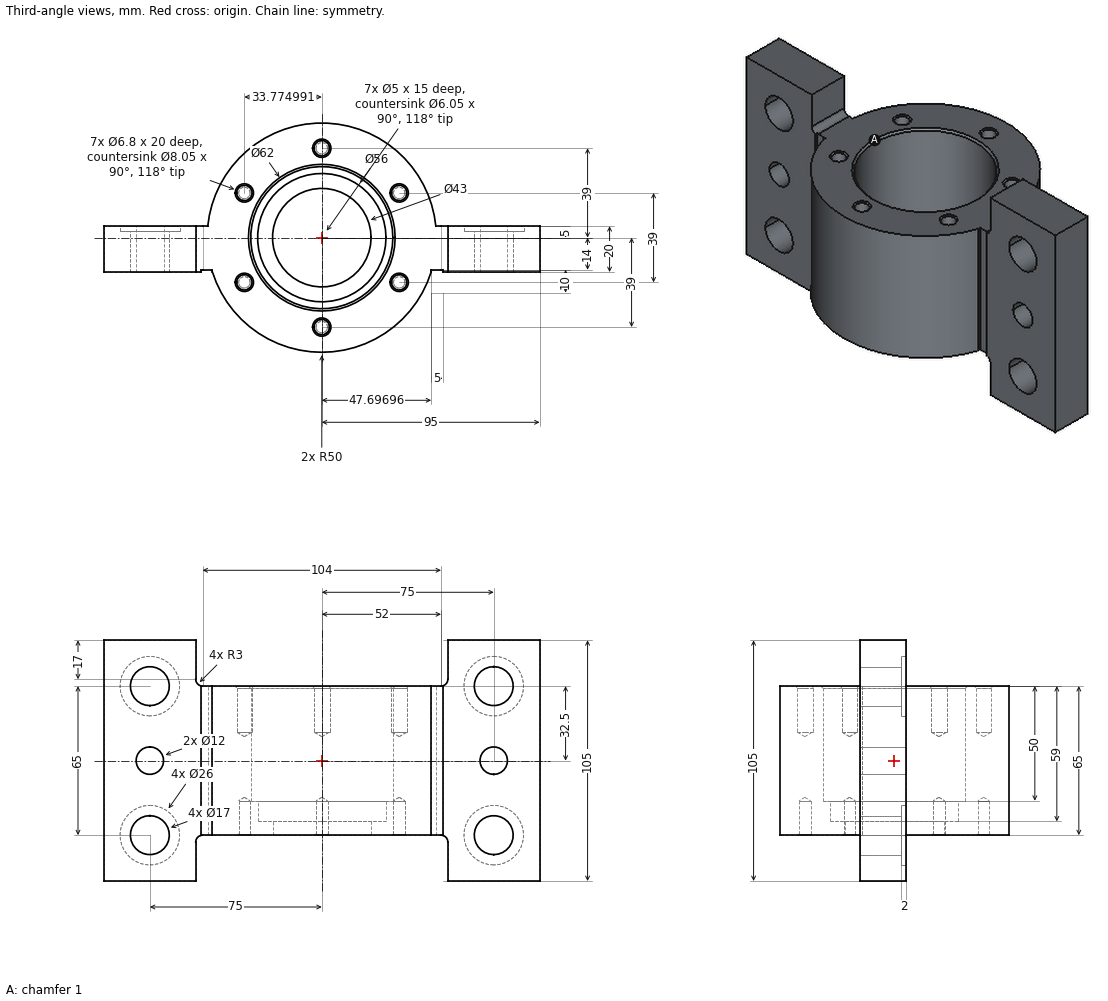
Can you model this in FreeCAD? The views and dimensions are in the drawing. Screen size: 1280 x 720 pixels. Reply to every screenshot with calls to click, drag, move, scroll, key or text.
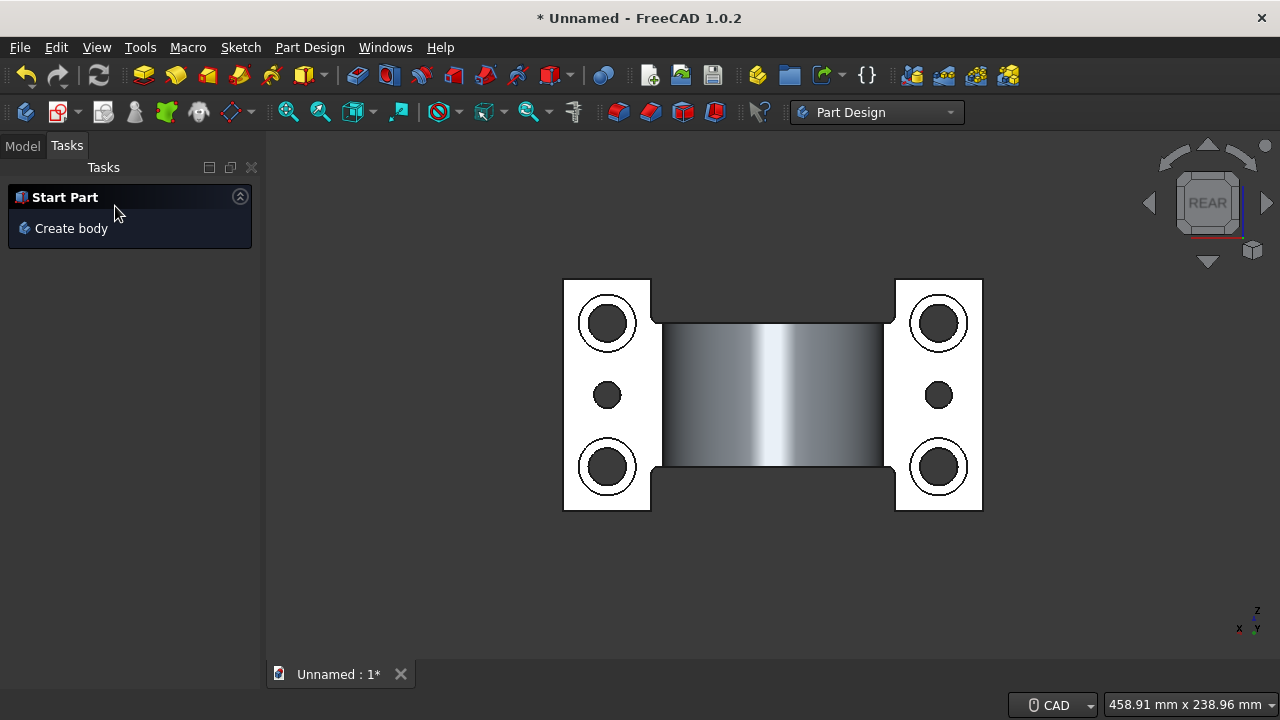
click(290, 112)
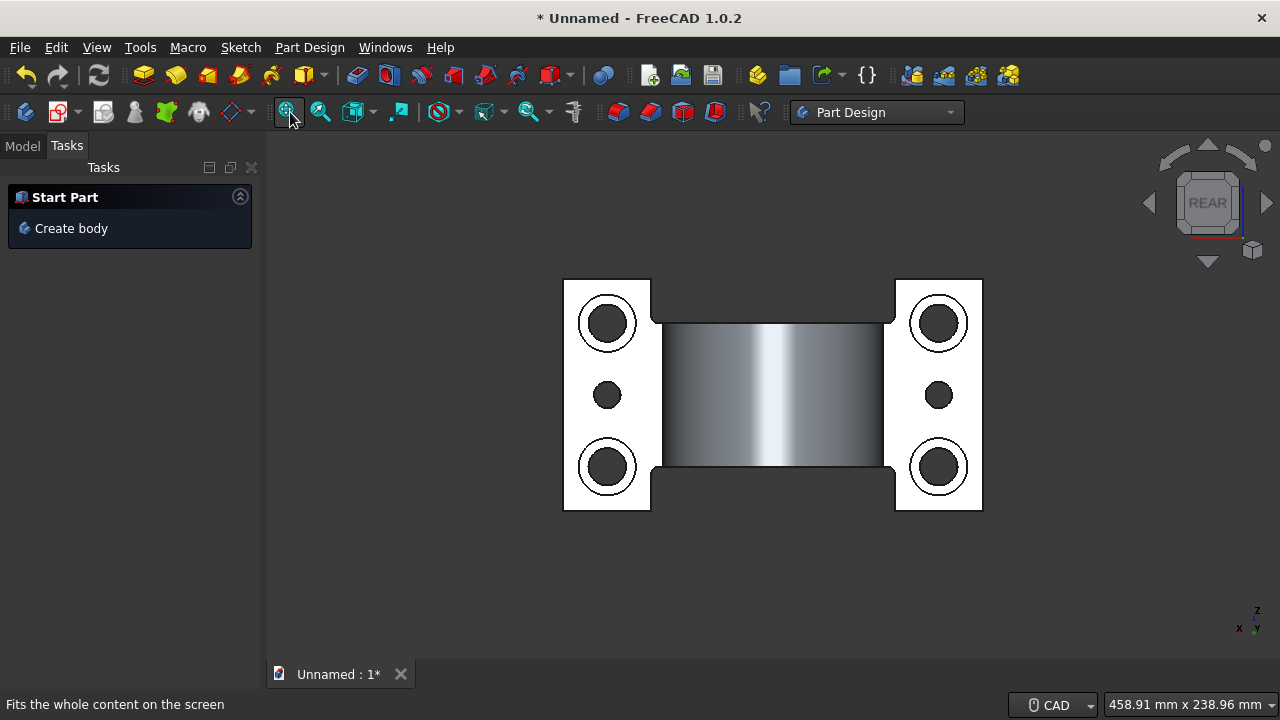
key(0)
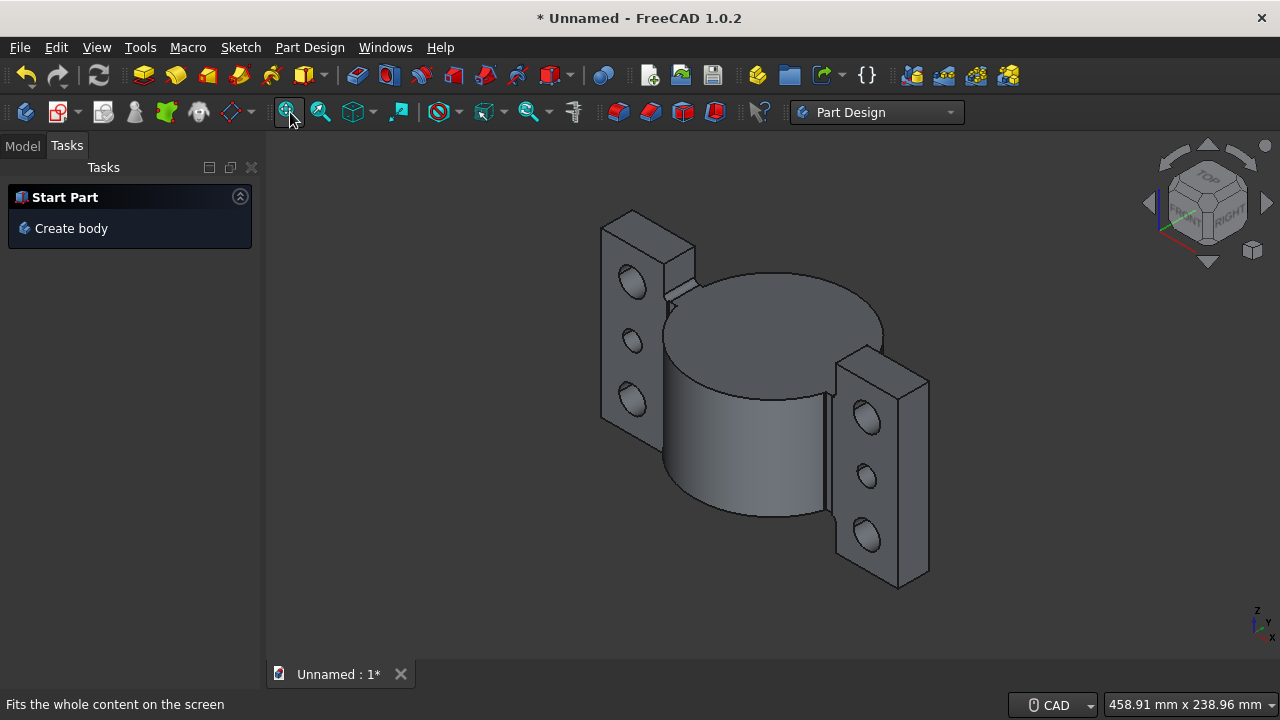
click(773, 335)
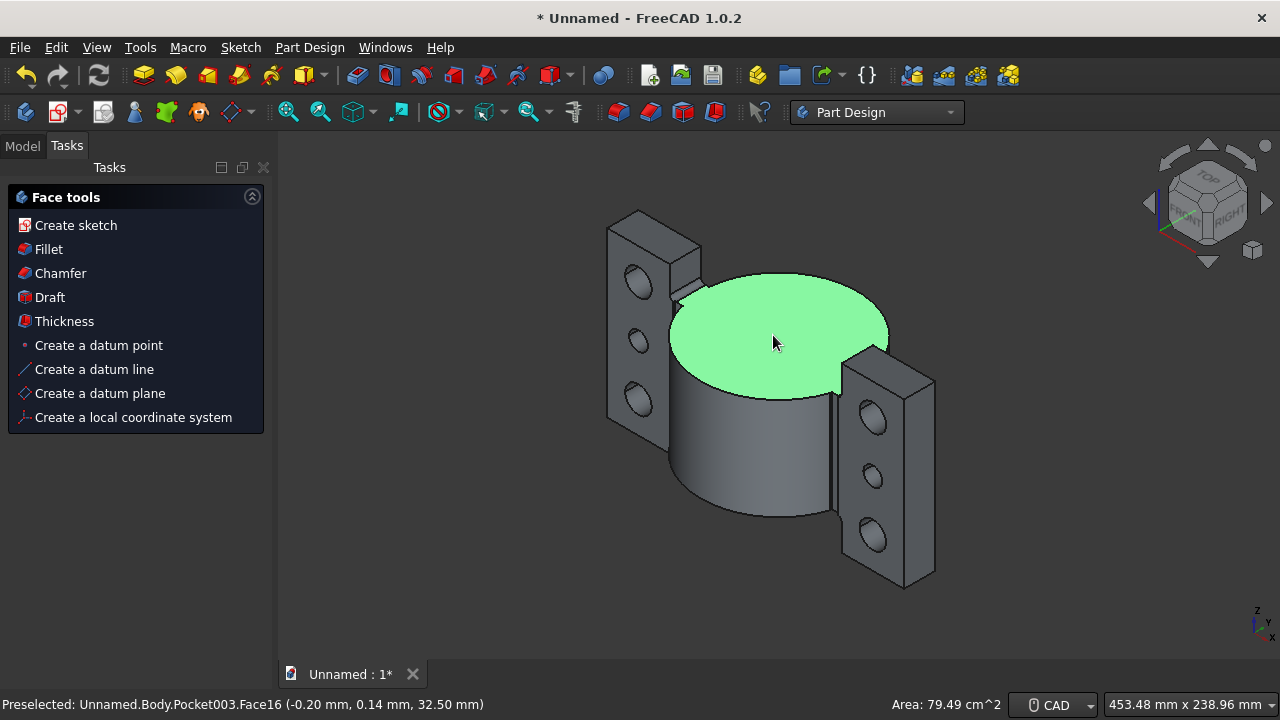
click(58, 112)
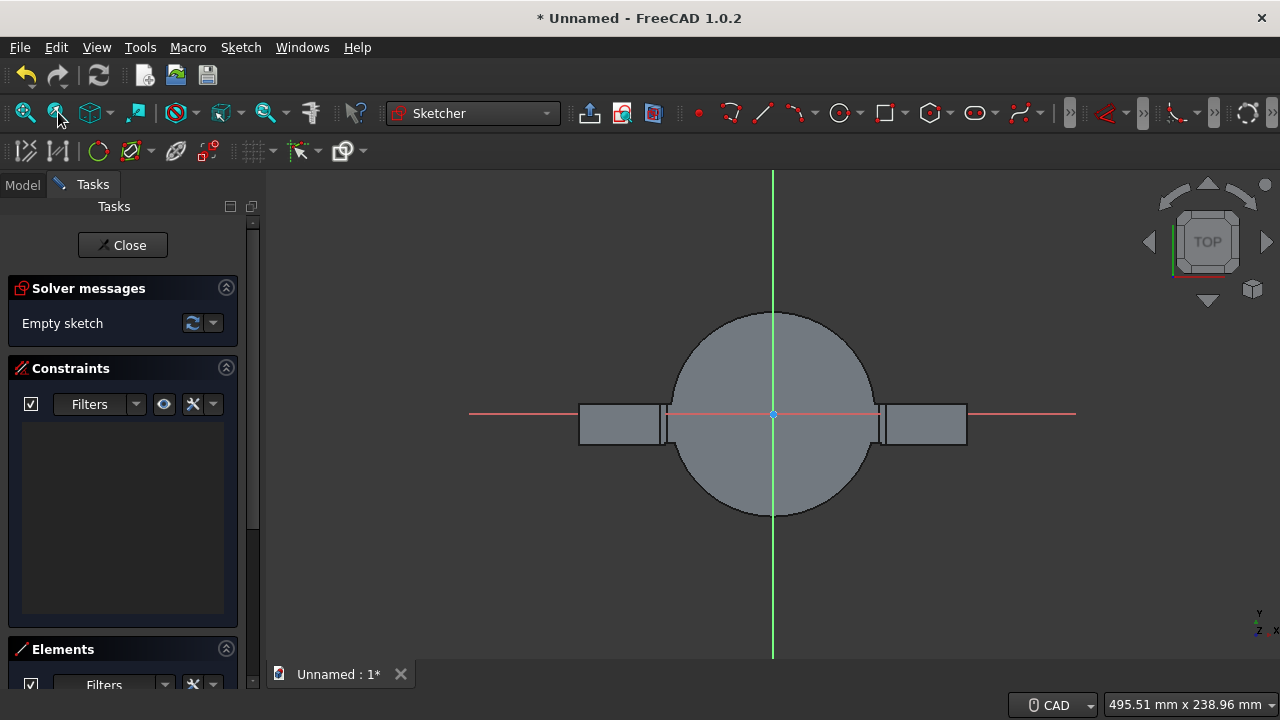
scroll(829, 414, up, 4)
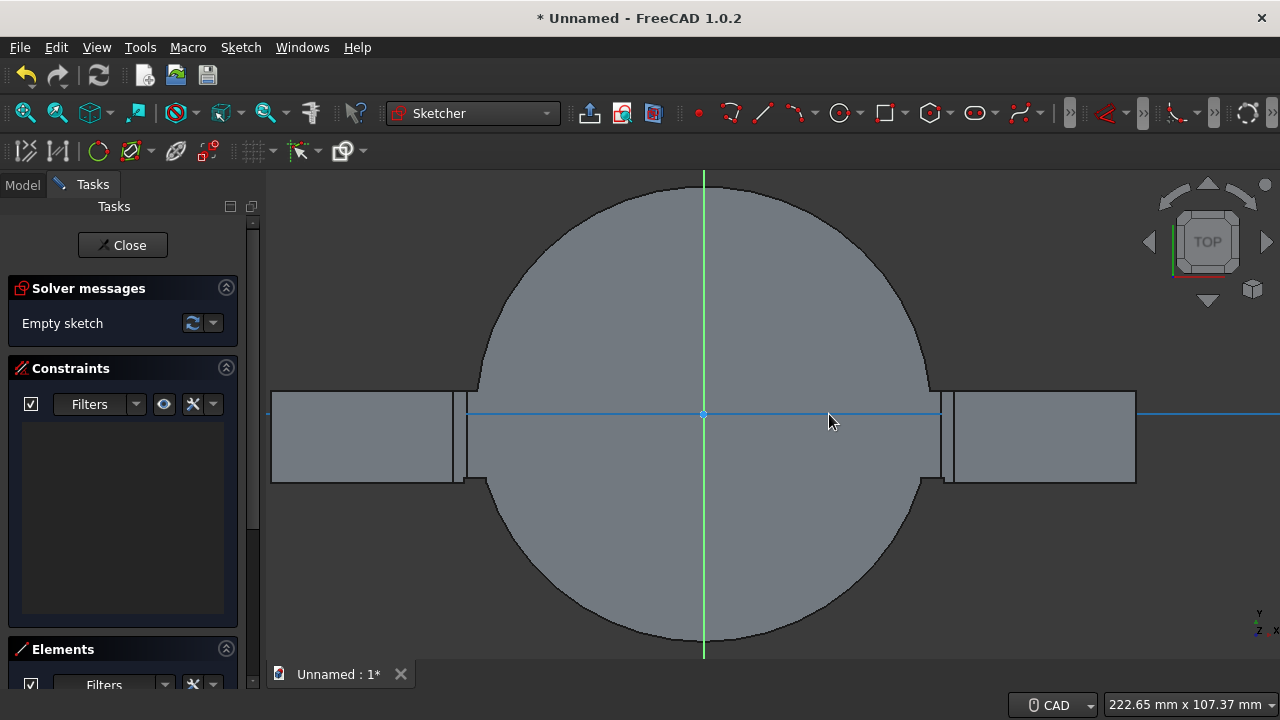
click(840, 114)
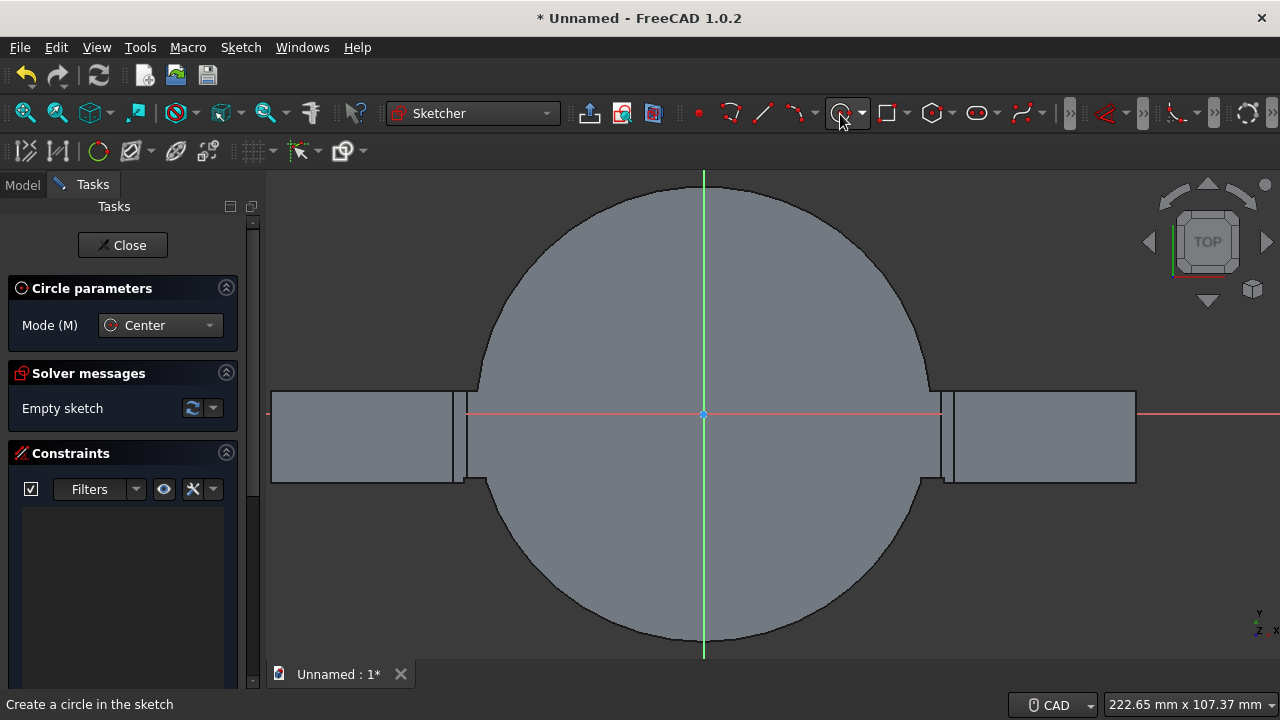
click(704, 414)
click(804, 314)
key(Escape)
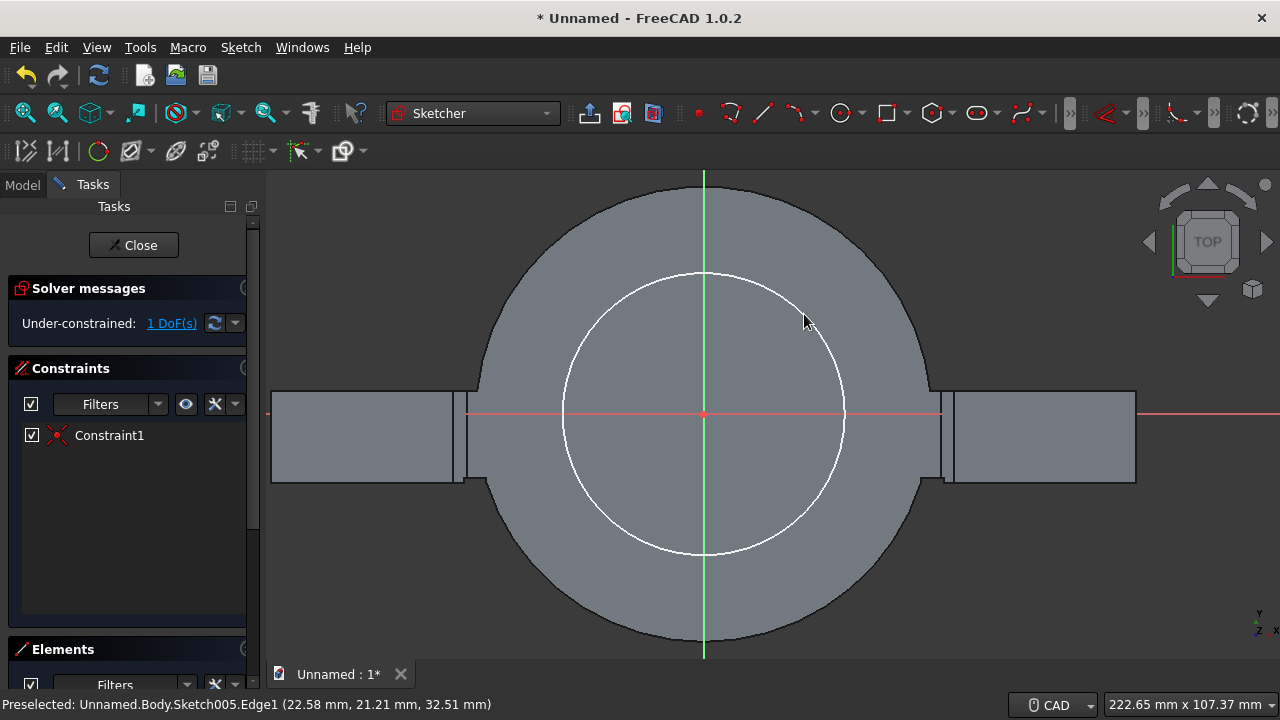
click(1106, 114)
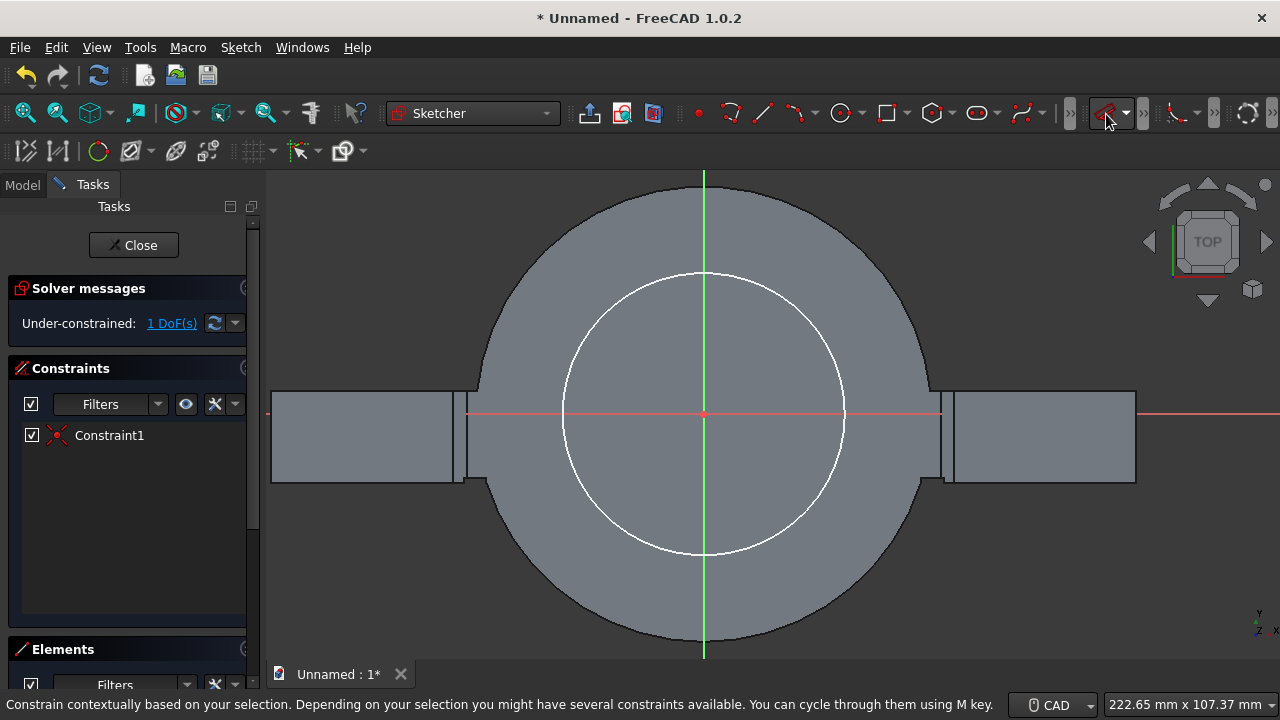
click(803, 314)
click(826, 291)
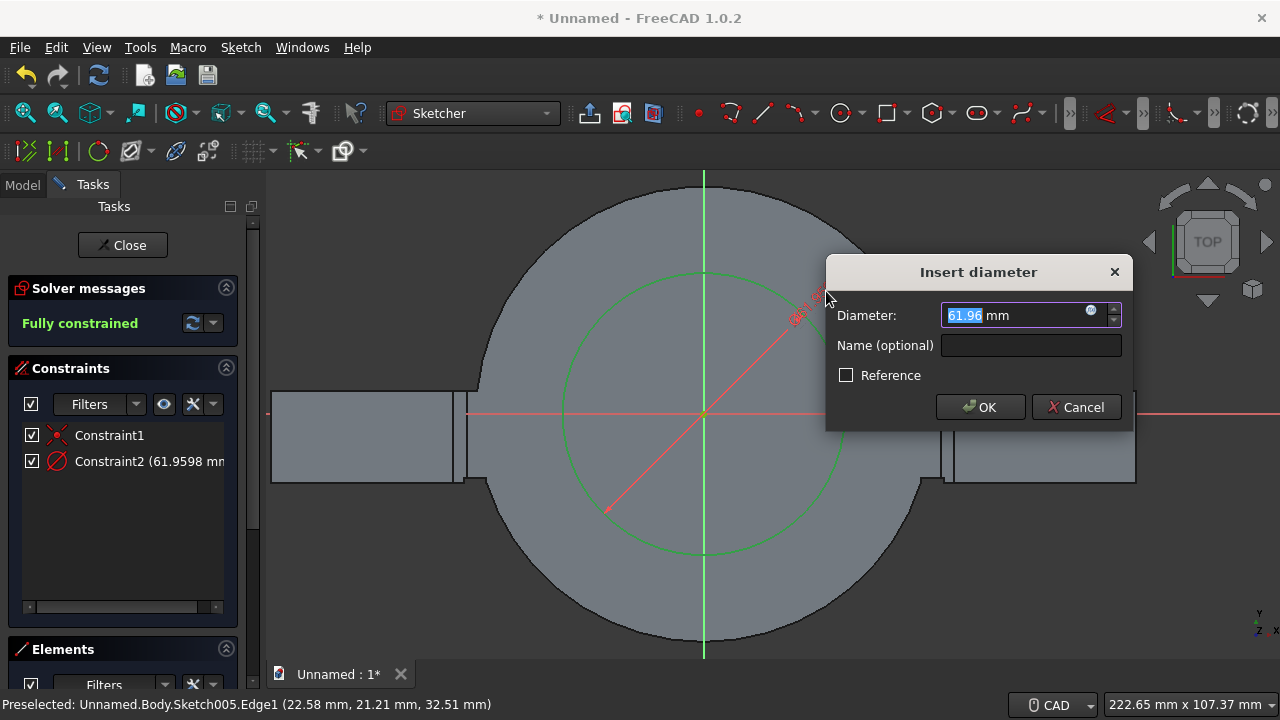
text(62)
key(Return)
key(Escape)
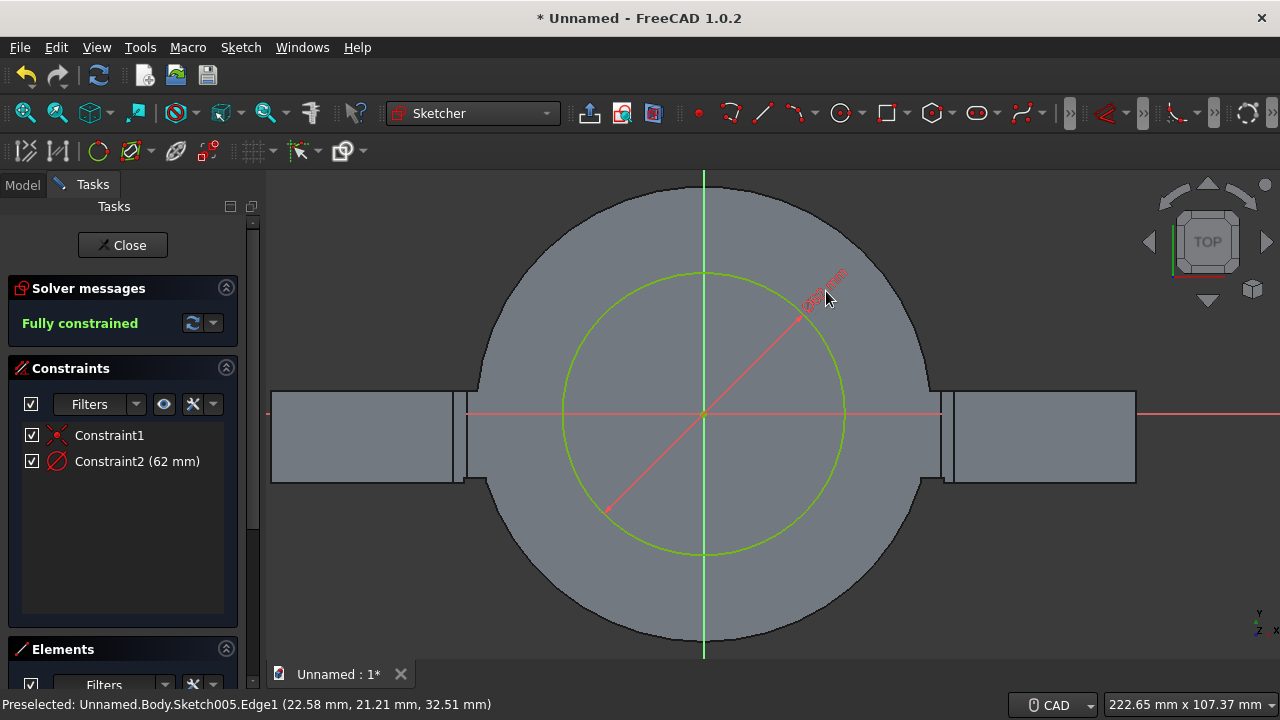
click(123, 245)